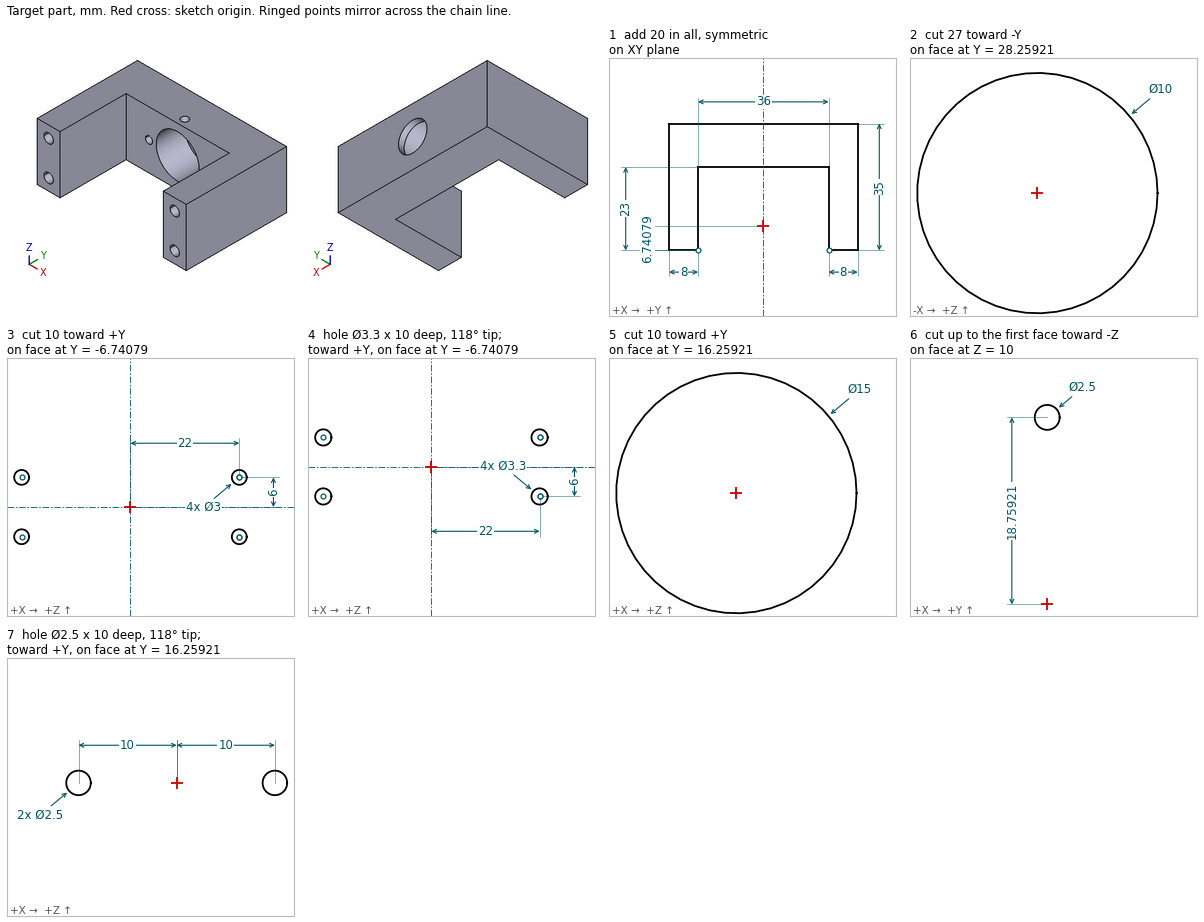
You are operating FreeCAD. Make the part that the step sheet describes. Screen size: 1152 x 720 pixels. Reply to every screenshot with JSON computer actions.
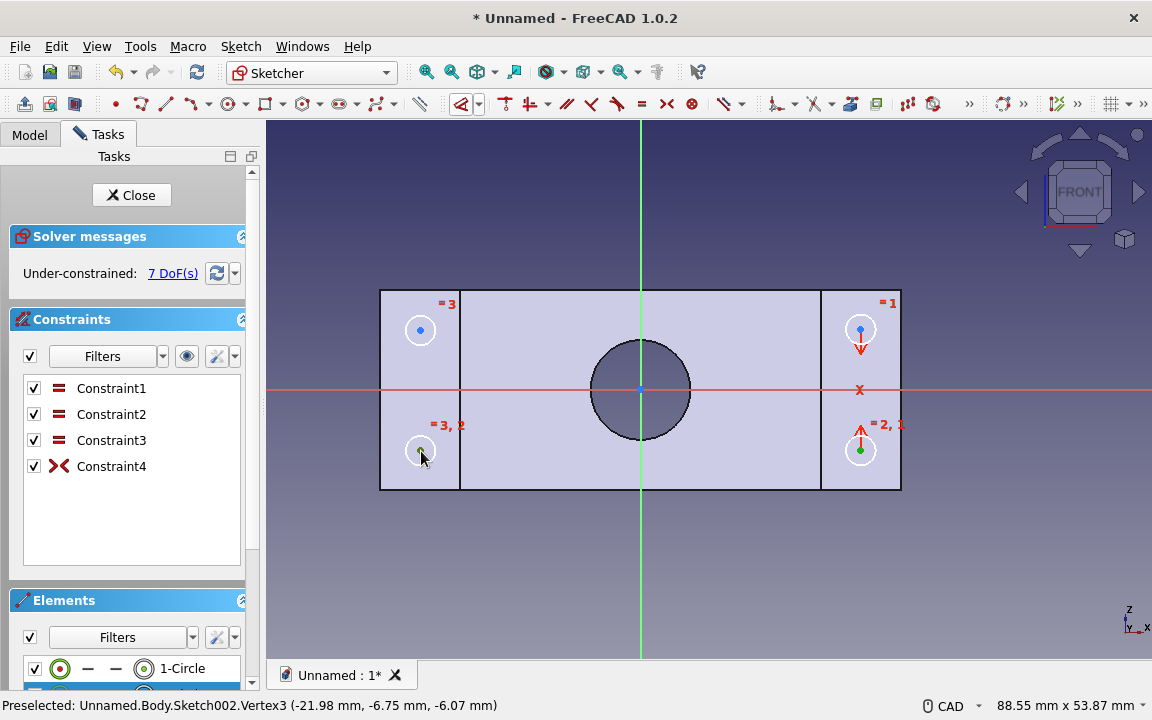
{"action": "left_click", "coordinate": [641, 596]}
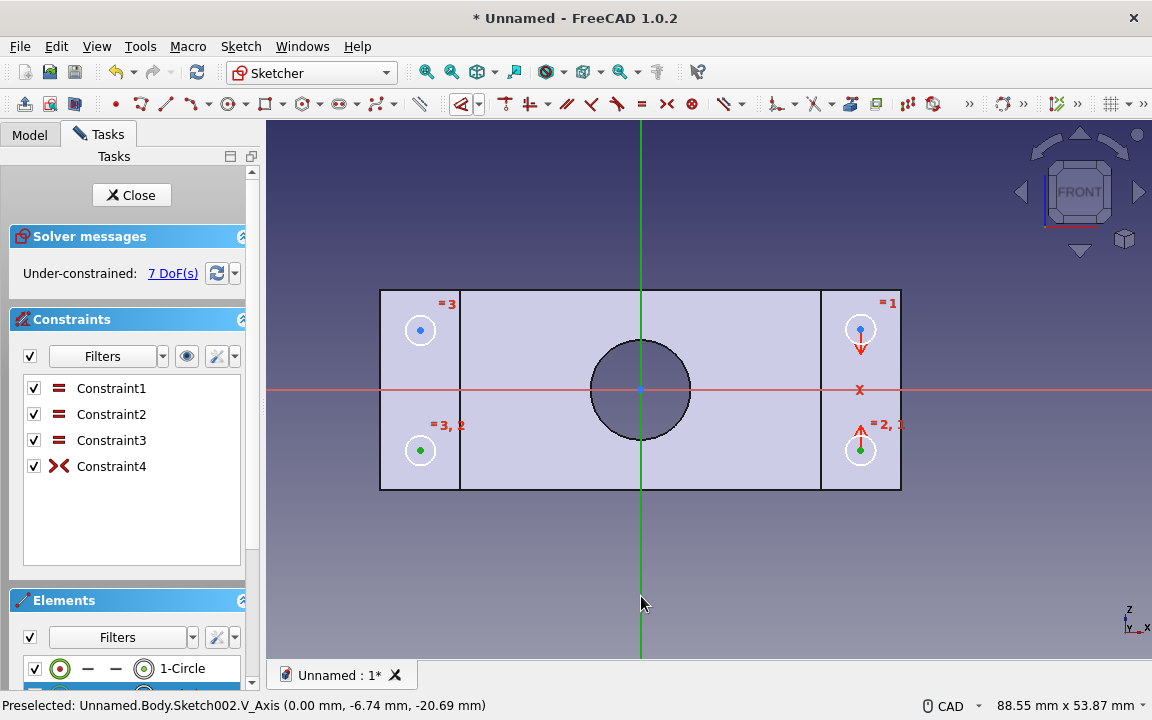
{"action": "left_click", "coordinate": [667, 104]}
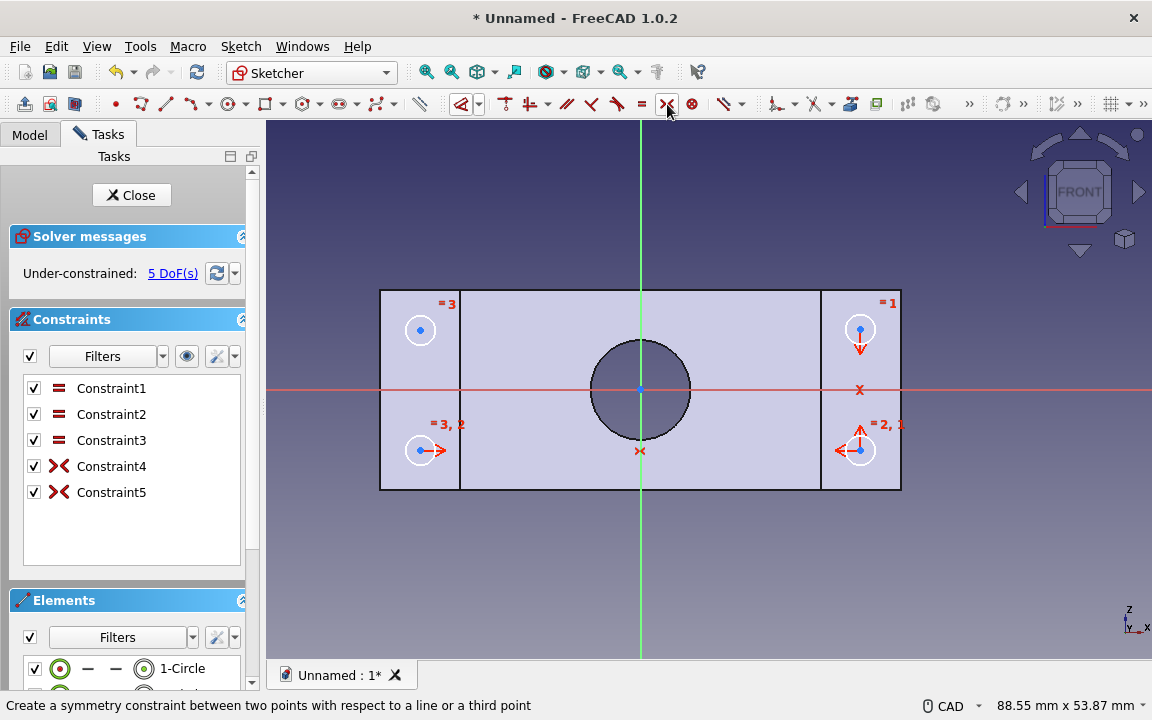
{"action": "left_click", "coordinate": [860, 329]}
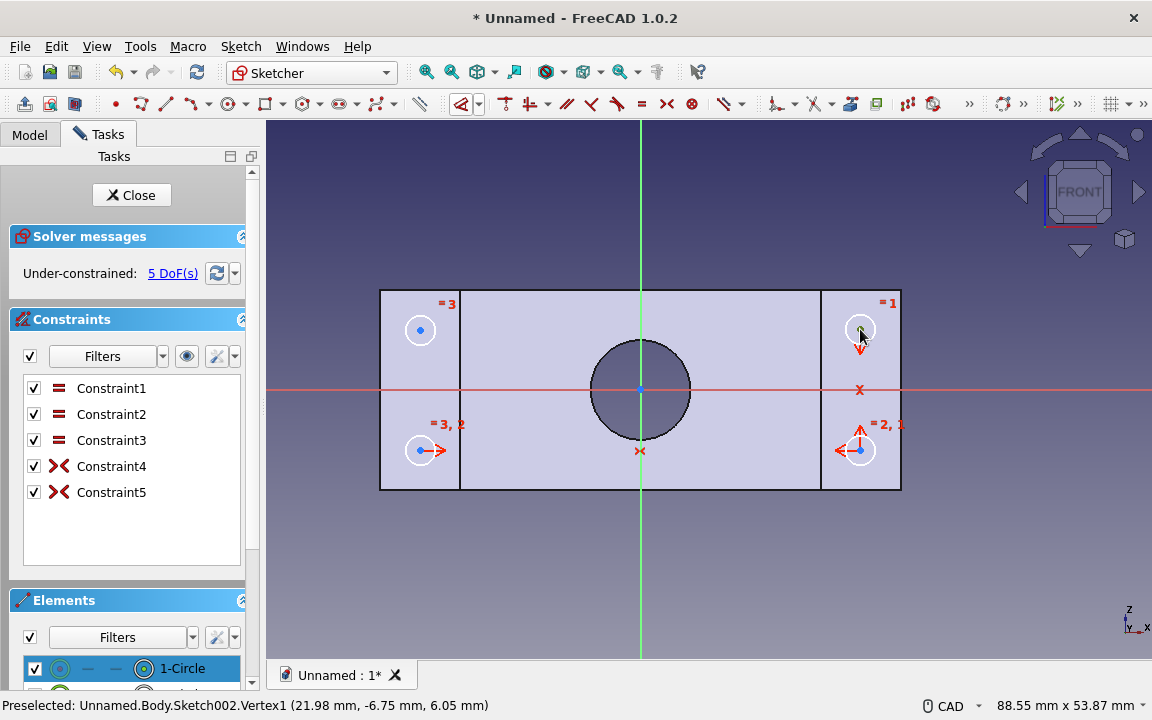
{"action": "left_click", "coordinate": [421, 331]}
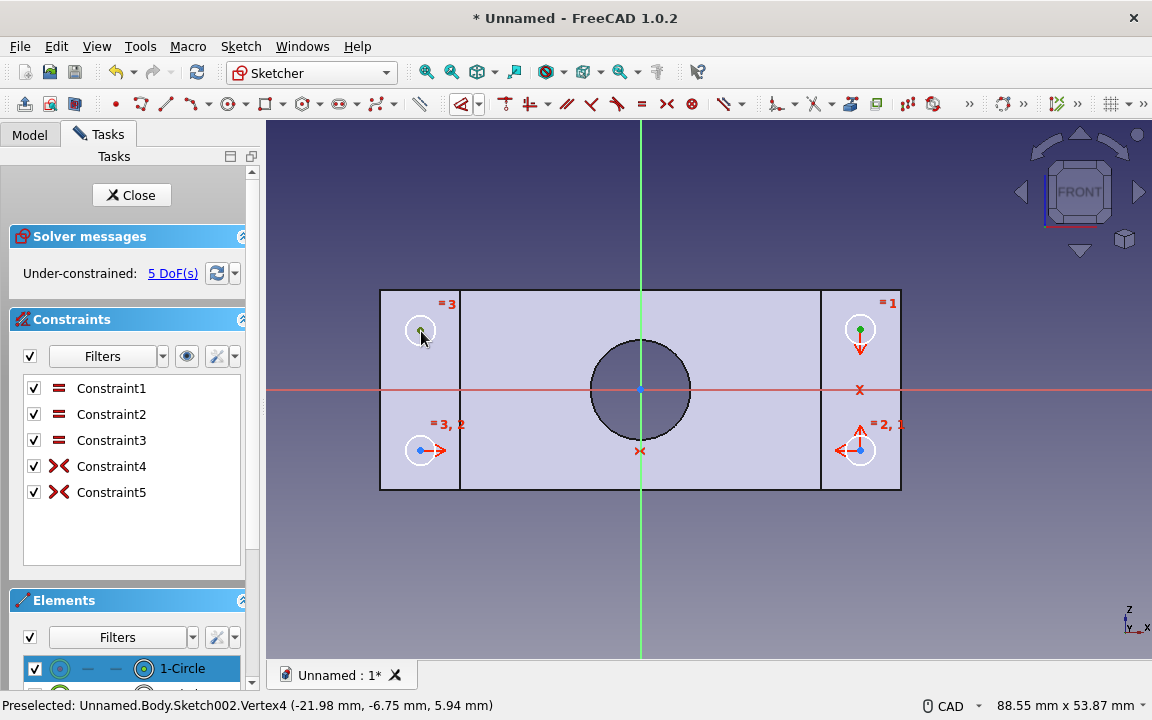
{"action": "left_click", "coordinate": [641, 596]}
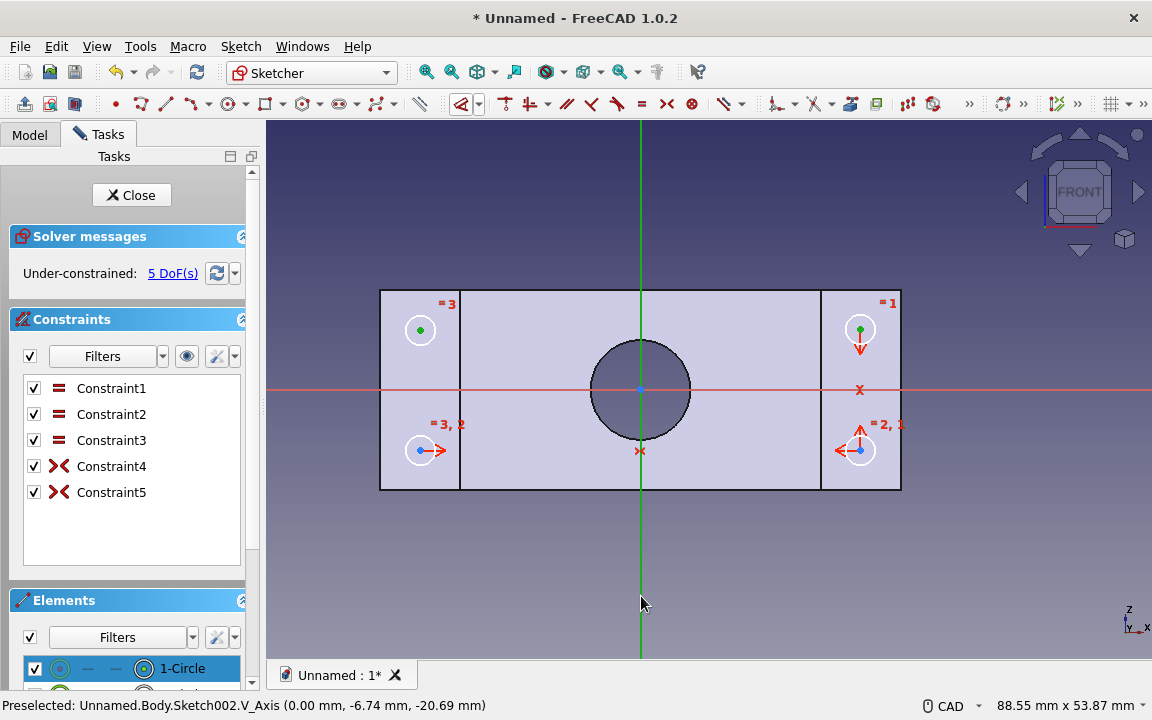
{"action": "left_click", "coordinate": [667, 104]}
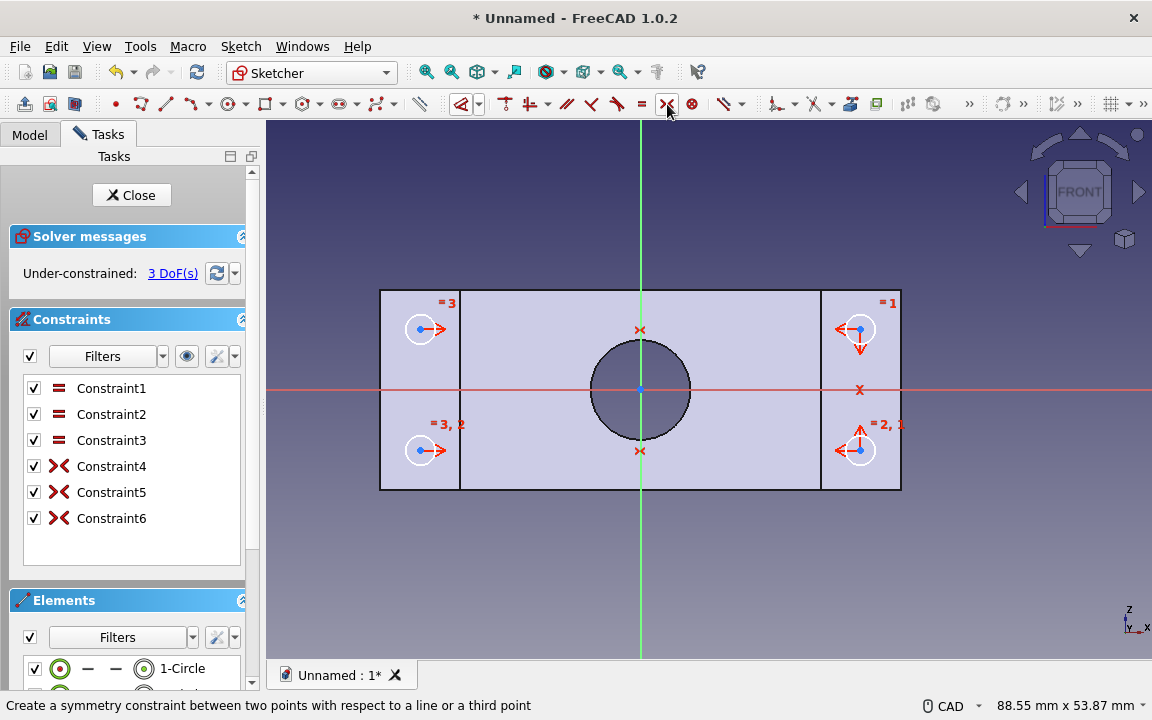
{"action": "scroll", "coordinate": [871, 319], "scroll_direction": "up", "scroll_amount": 2}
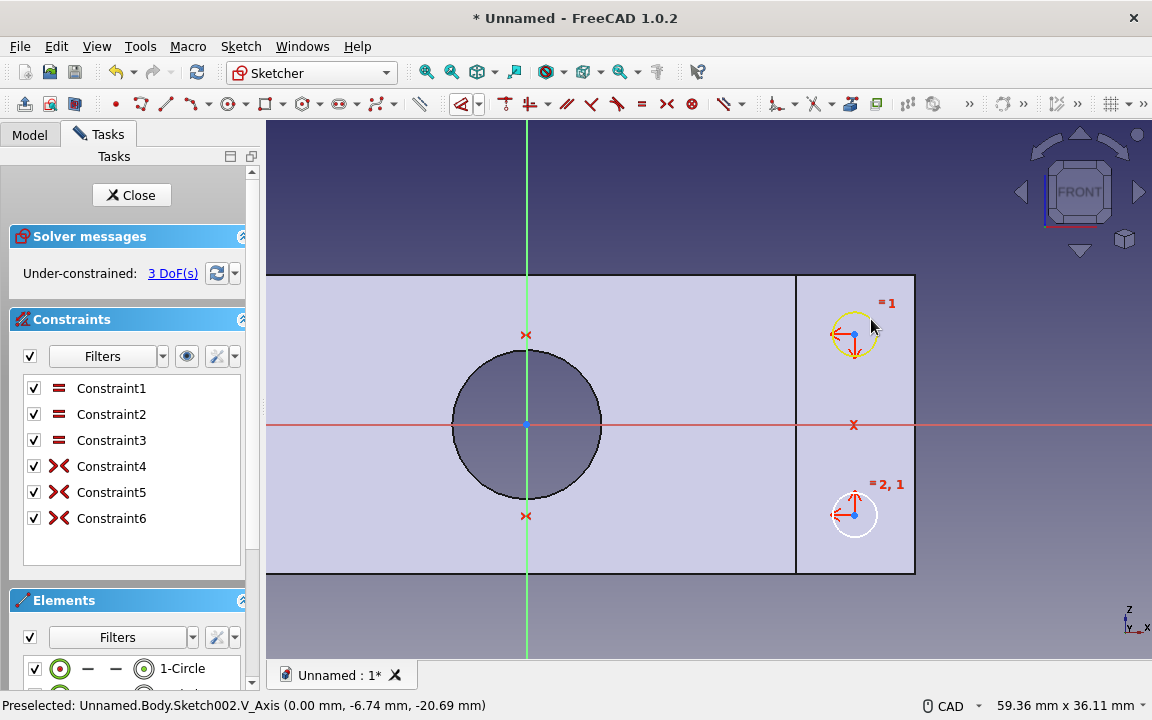
{"action": "left_click", "coordinate": [870, 319]}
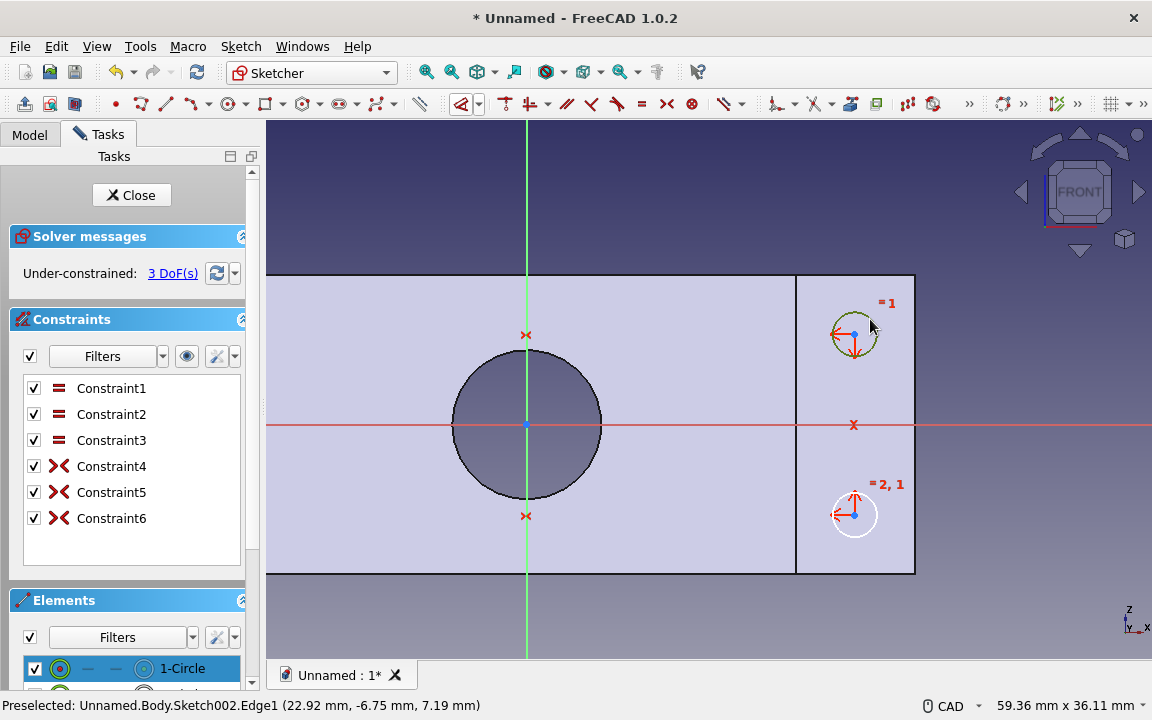
{"action": "key", "text": "k o"}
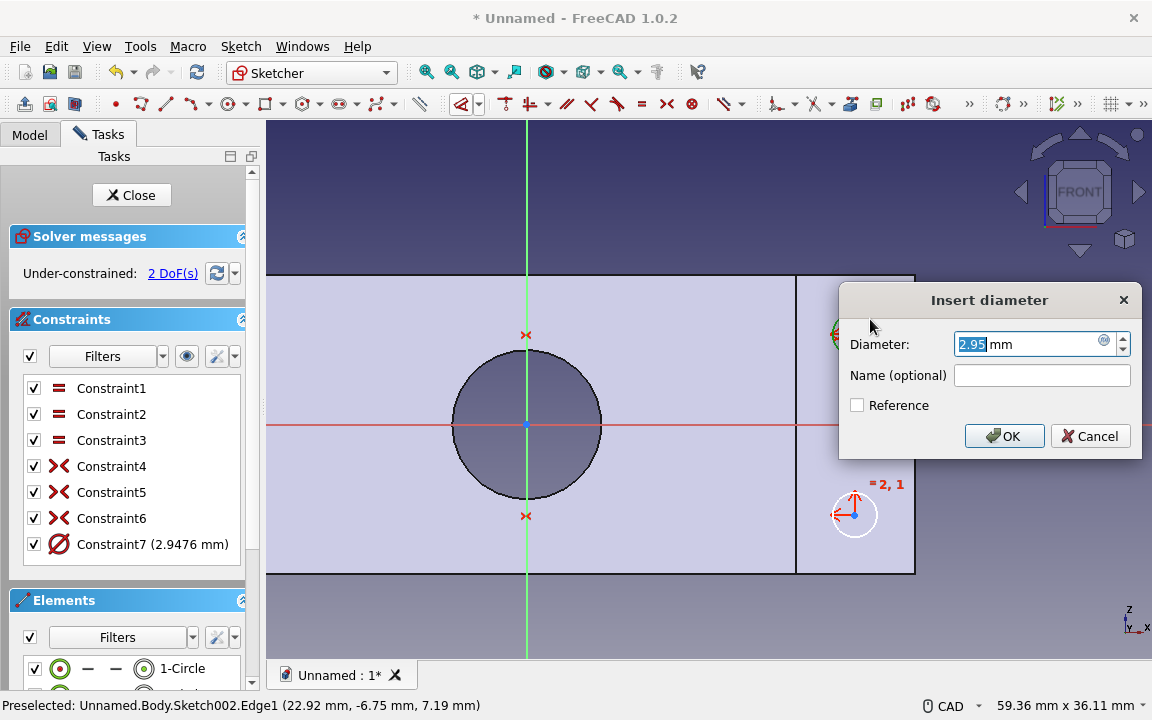
{"action": "type", "text": "3"}
{"action": "key", "text": "Return"}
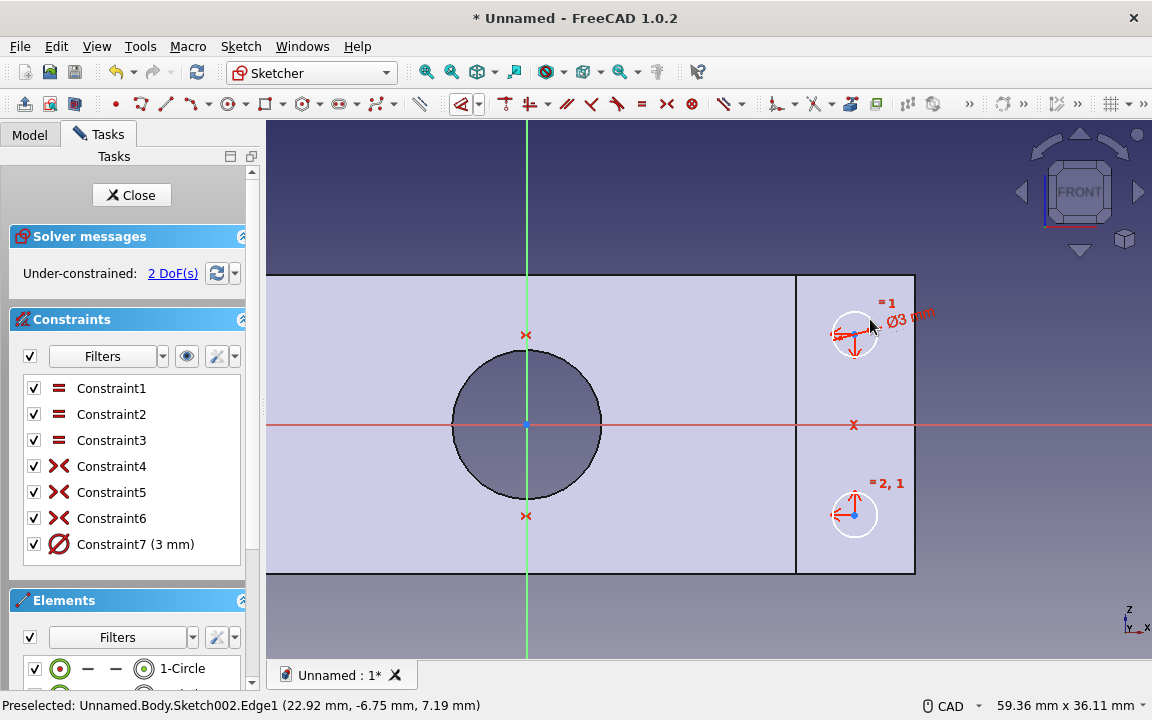
{"action": "left_click", "coordinate": [855, 334]}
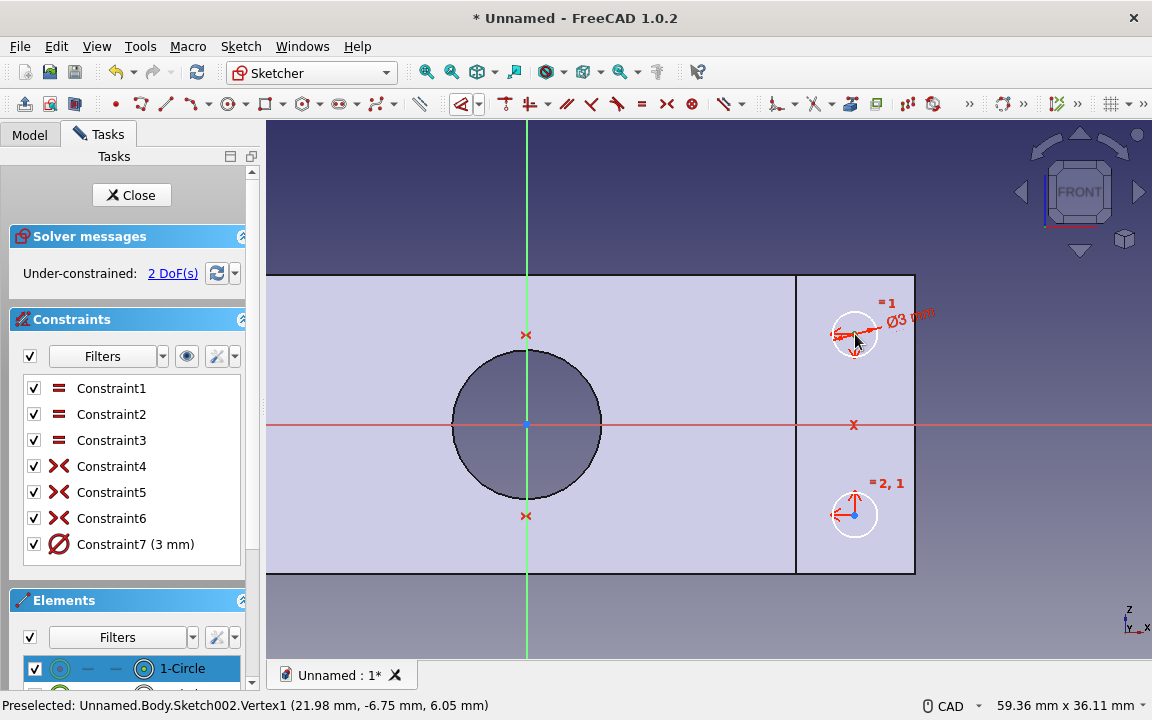
{"action": "key", "text": "i"}